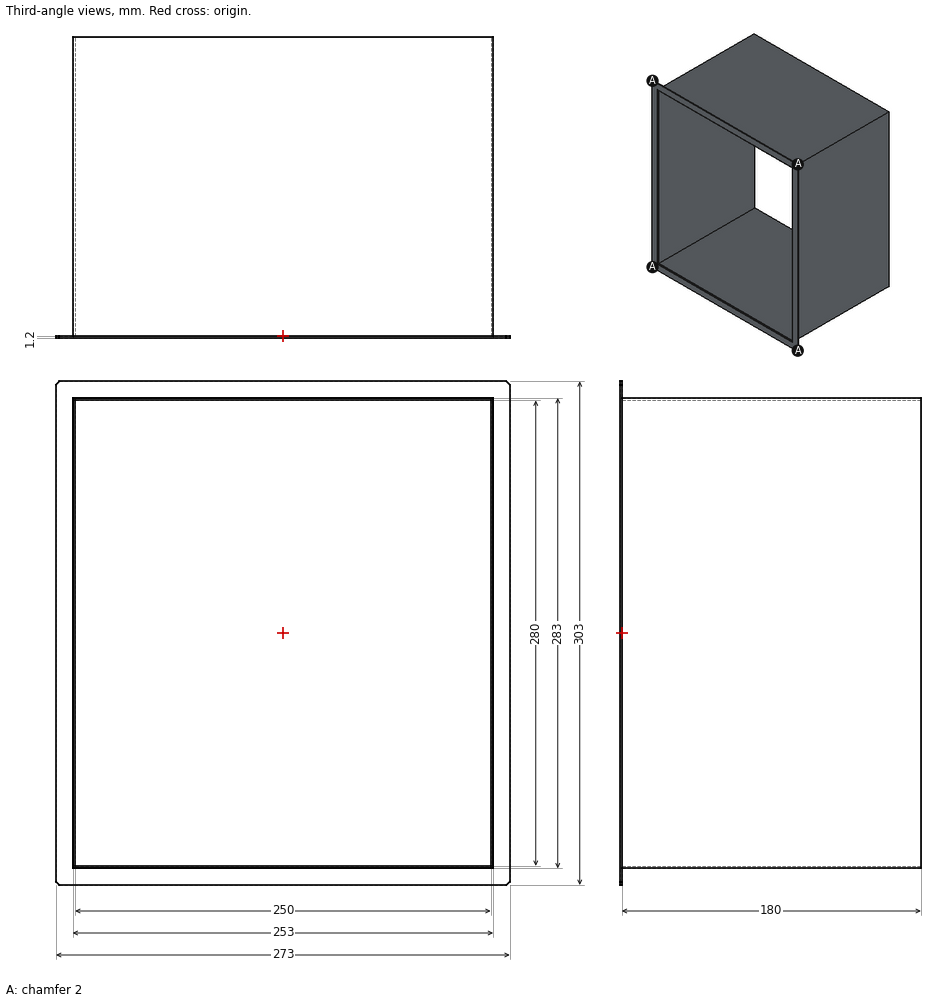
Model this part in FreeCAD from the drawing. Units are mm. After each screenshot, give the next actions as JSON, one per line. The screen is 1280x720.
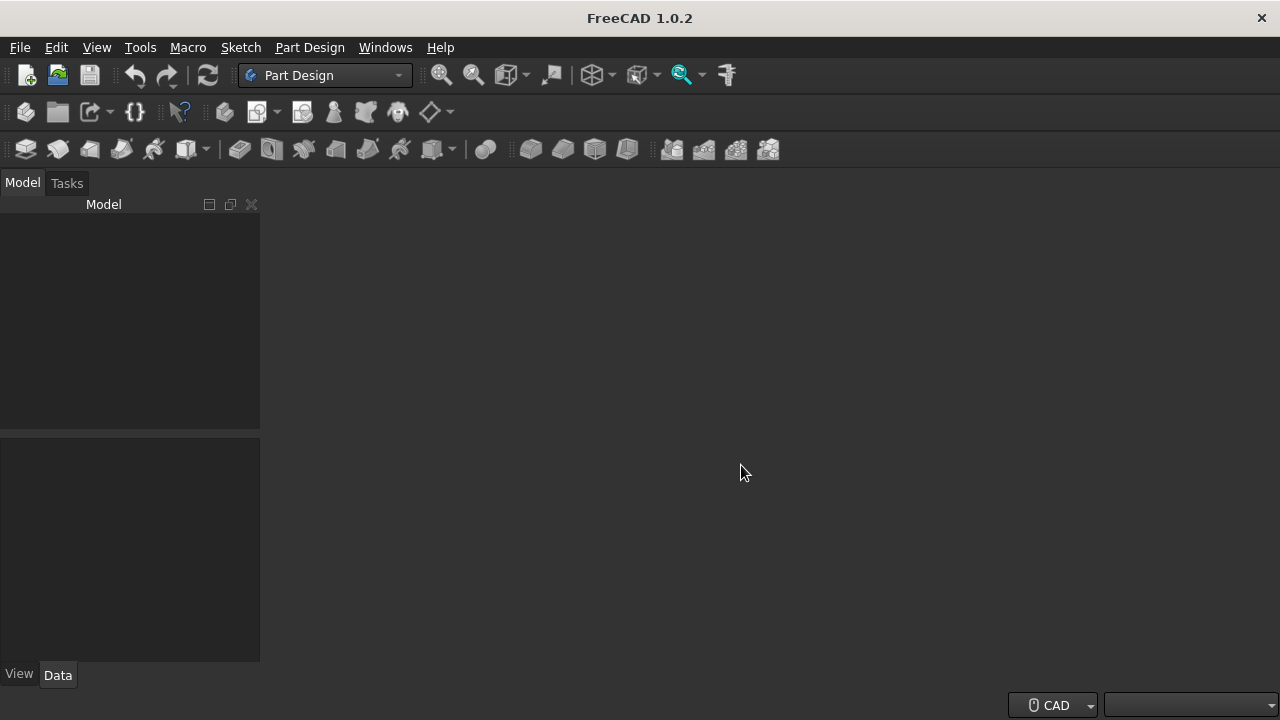
{"action": "key", "text": "ctrl+n"}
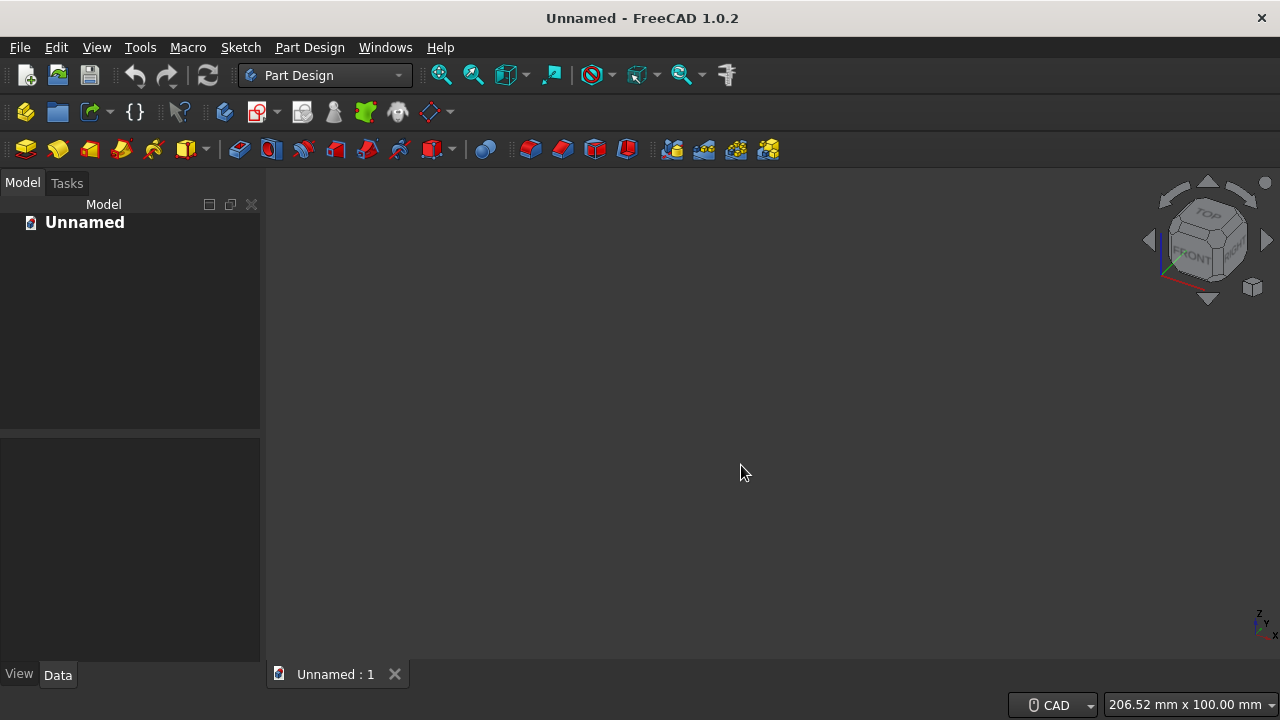
{"action": "left_click", "coordinate": [258, 112]}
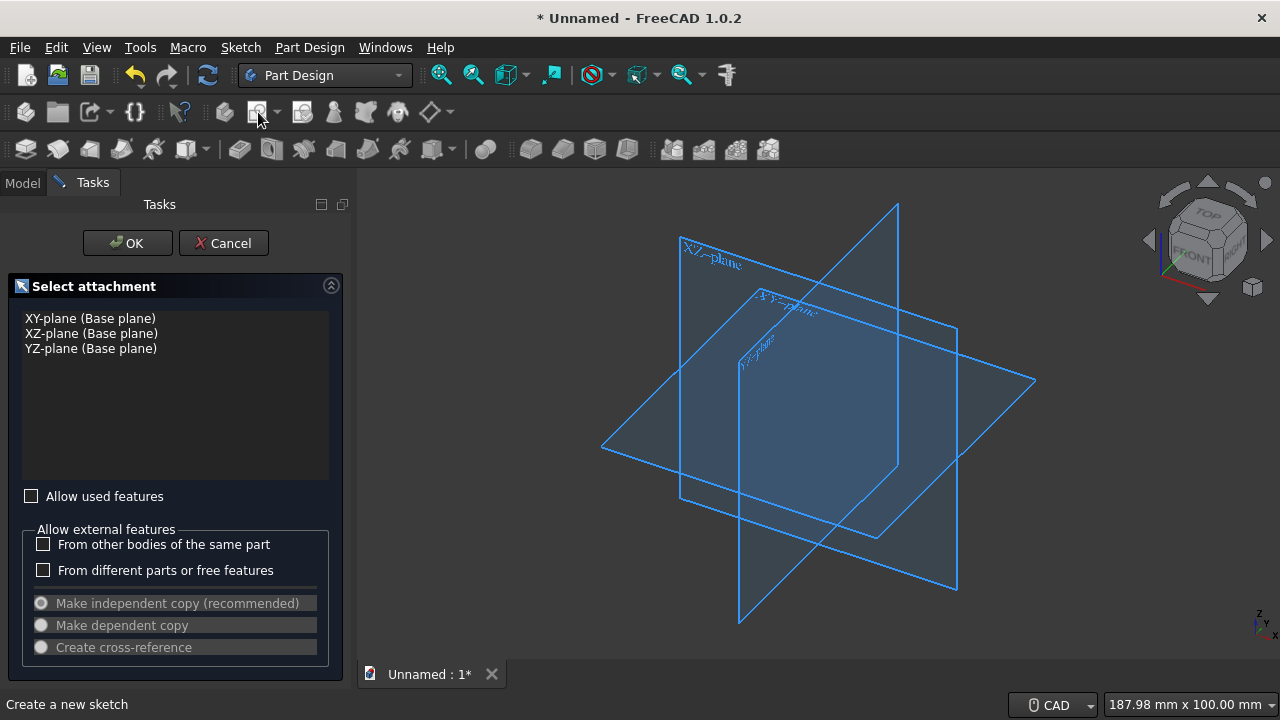
{"action": "left_click", "coordinate": [82, 334]}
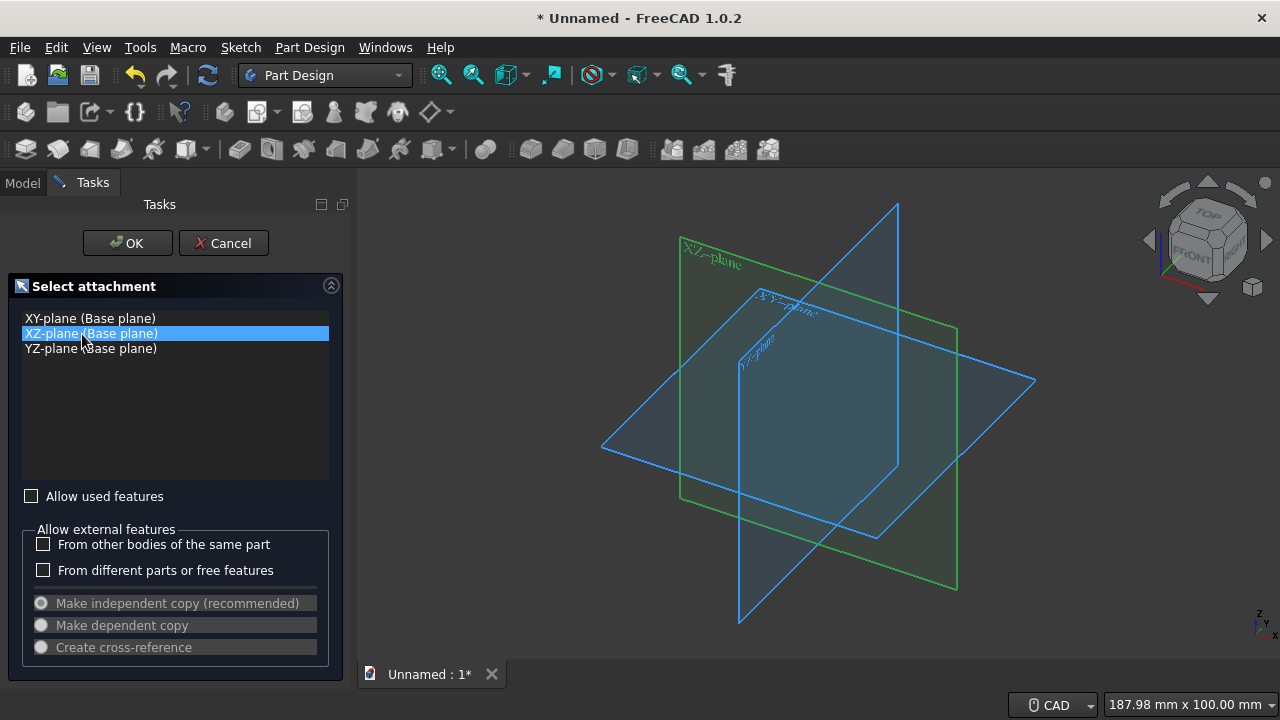
{"action": "left_click", "coordinate": [128, 243]}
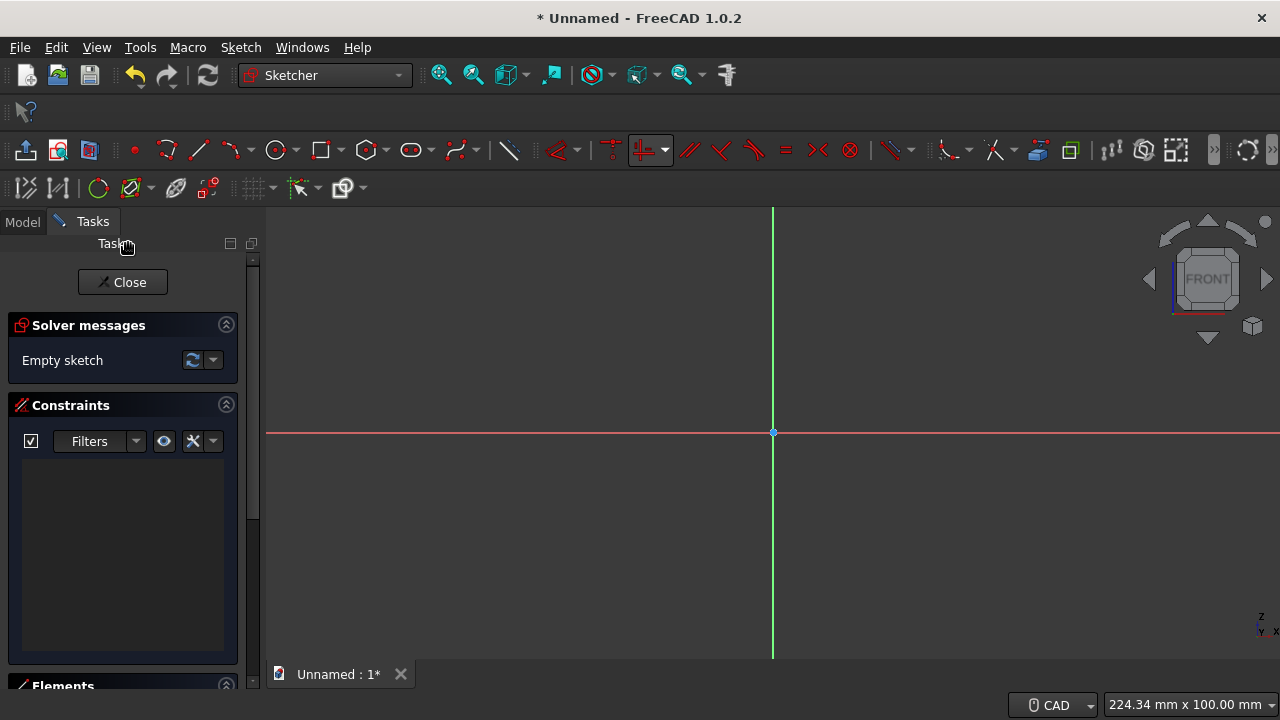
{"action": "scroll", "coordinate": [687, 433], "scroll_direction": "down", "scroll_amount": 8}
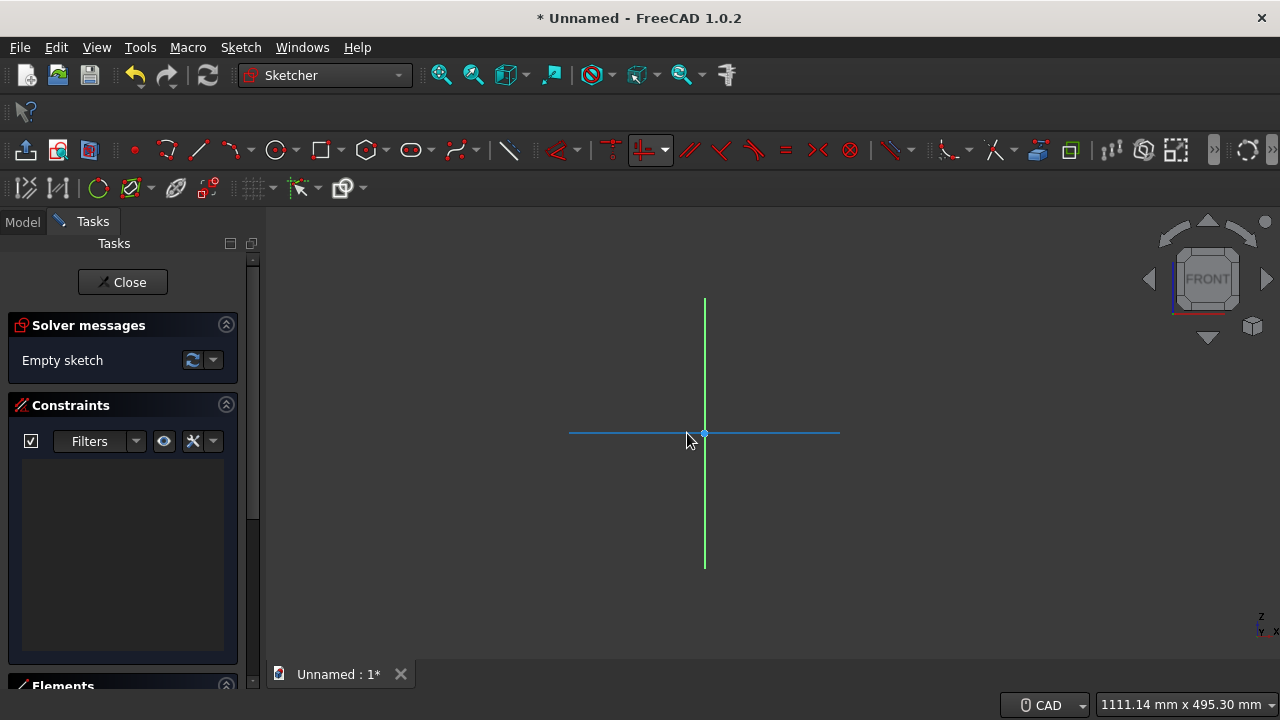
{"action": "key", "text": "g v"}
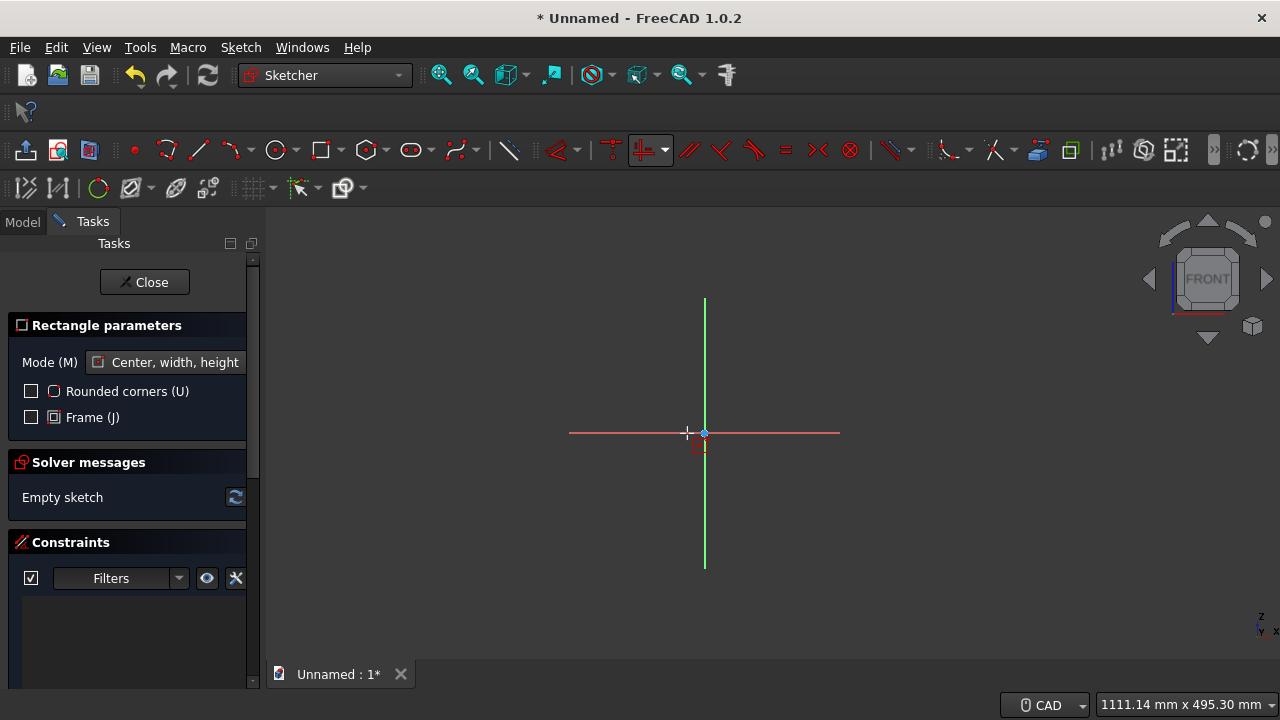
{"action": "left_click", "coordinate": [705, 433]}
{"action": "left_click", "coordinate": [820, 304]}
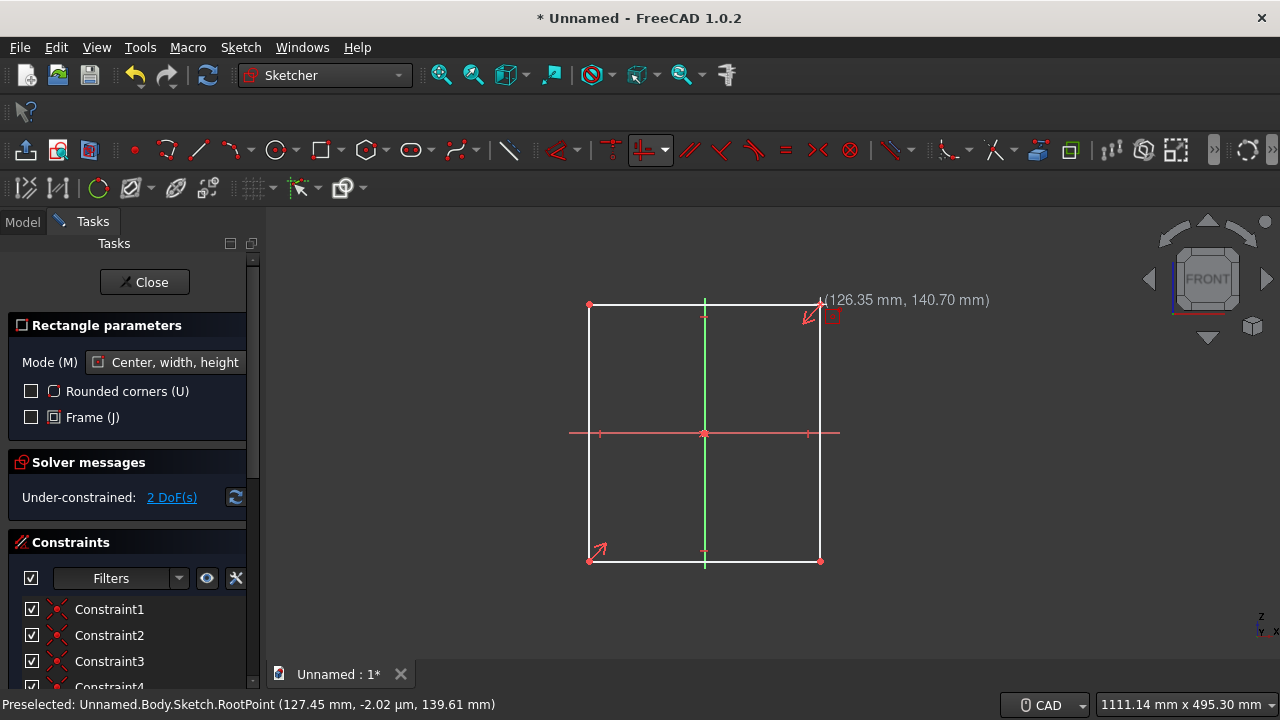
{"action": "left_click", "coordinate": [705, 433]}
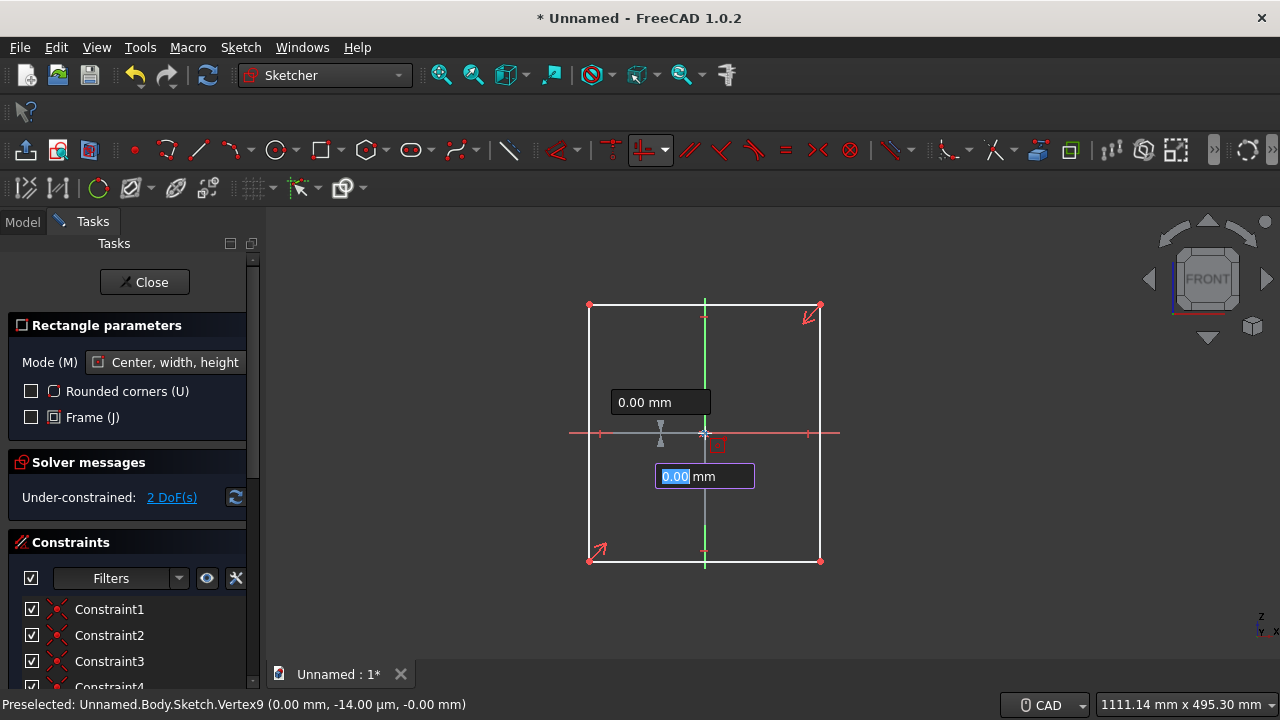
{"action": "scroll", "coordinate": [819, 306], "scroll_direction": "up", "scroll_amount": 13}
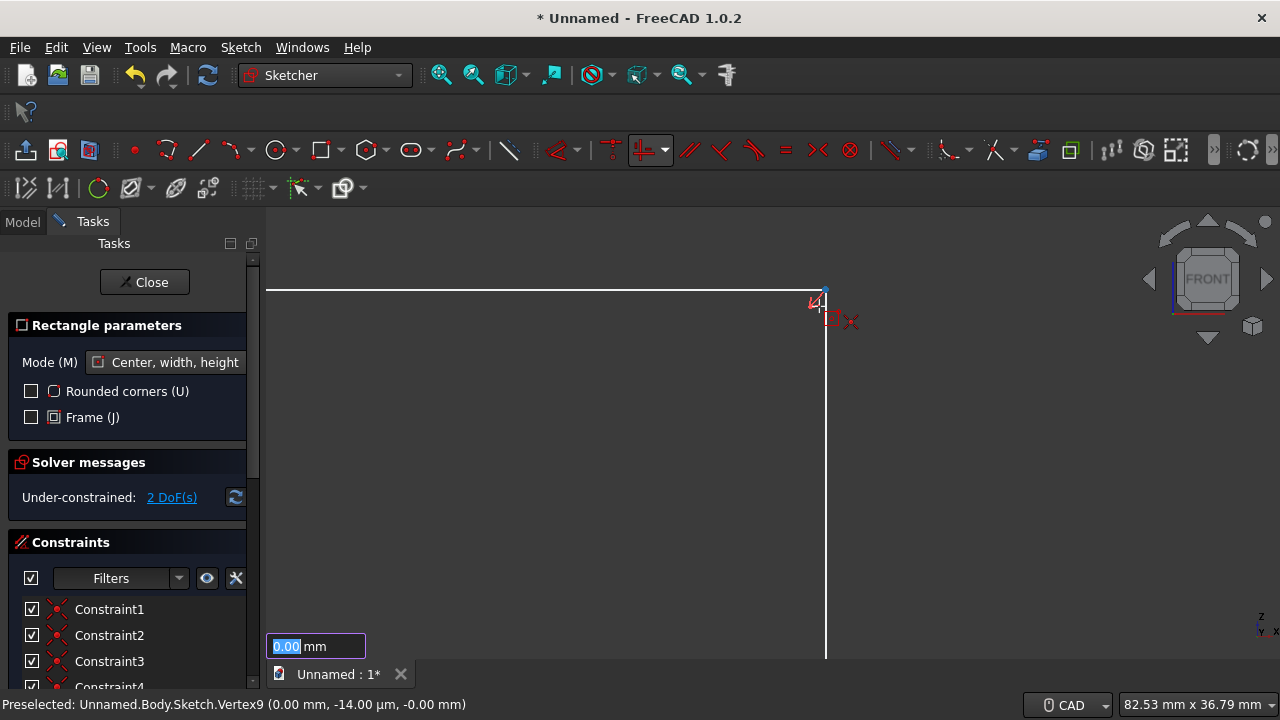
{"action": "left_click", "coordinate": [809, 298]}
{"action": "key", "text": "Escape"}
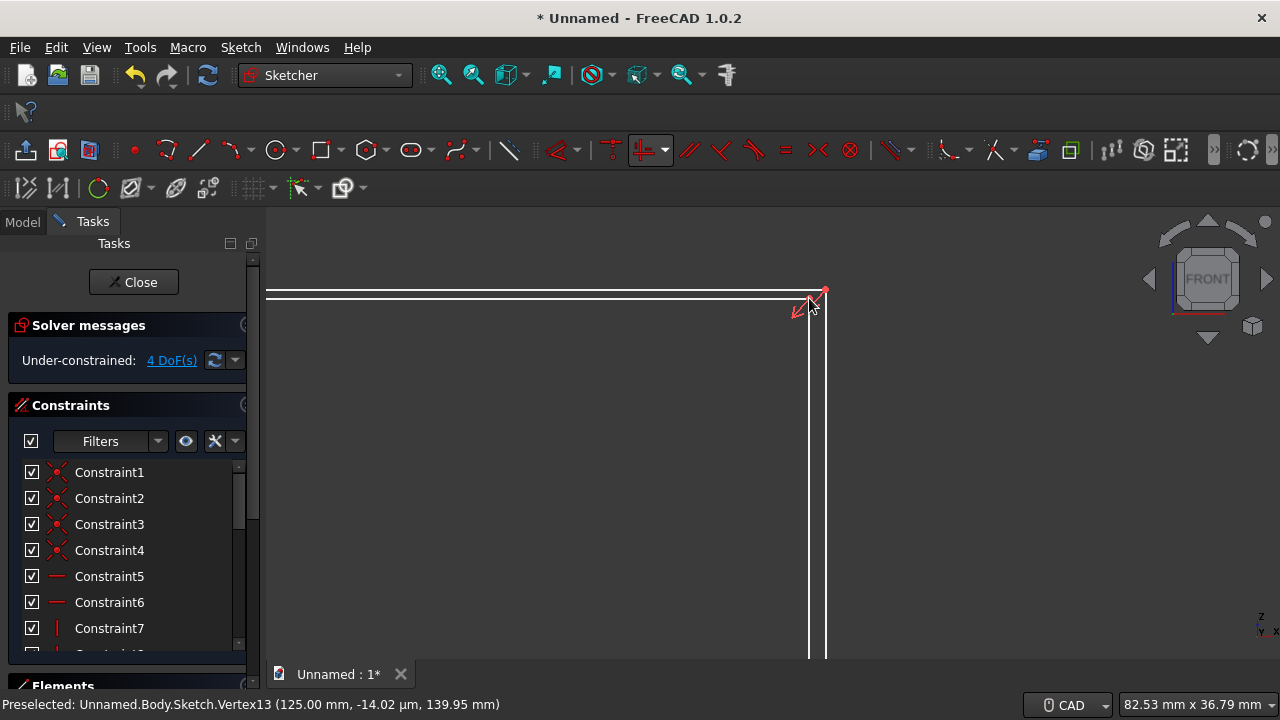
{"action": "key", "text": "d"}